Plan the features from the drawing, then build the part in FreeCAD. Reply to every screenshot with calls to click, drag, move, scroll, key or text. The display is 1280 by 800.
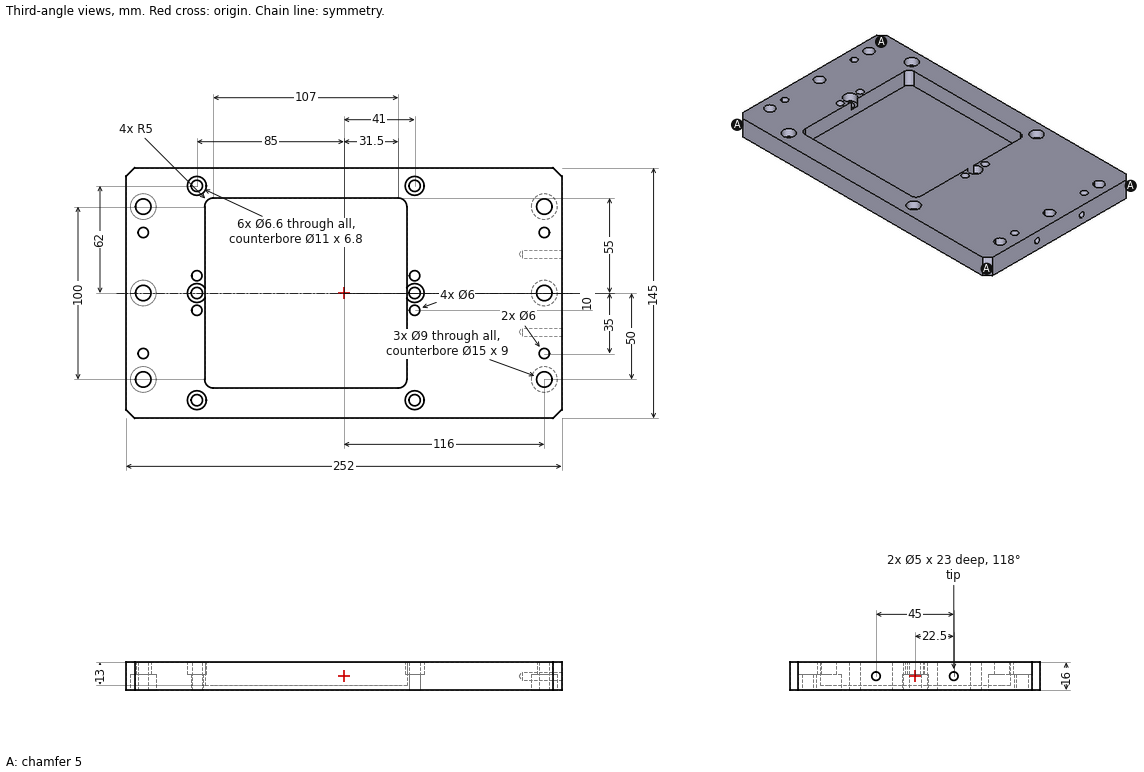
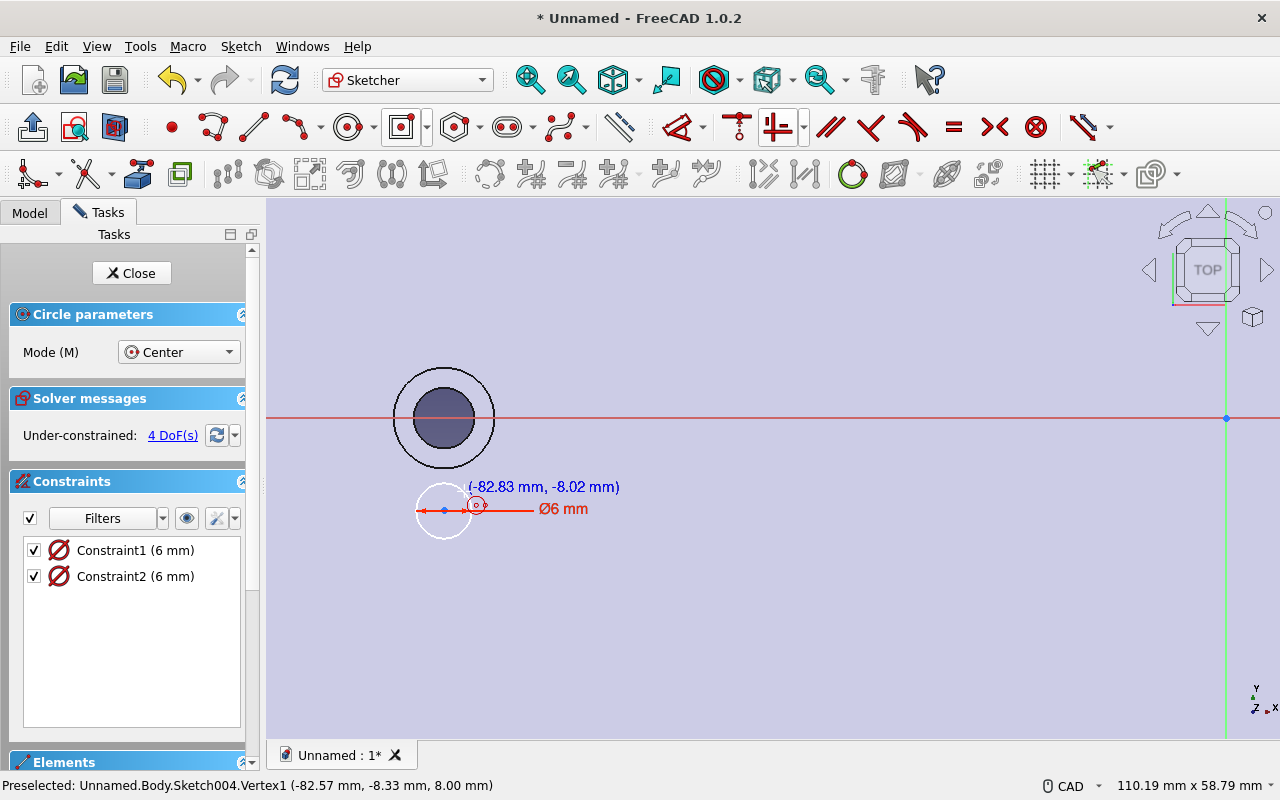
click(444, 326)
move(464, 307)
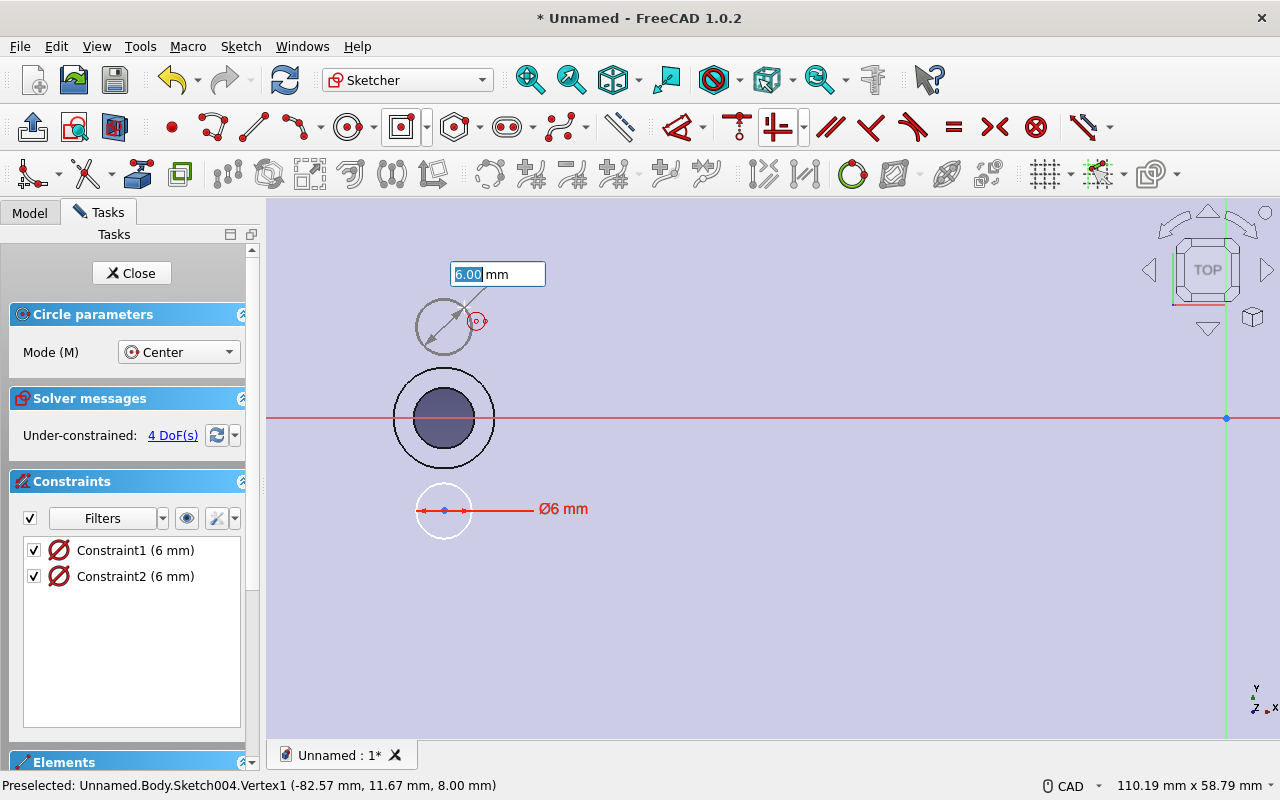
text(6)
key(Return)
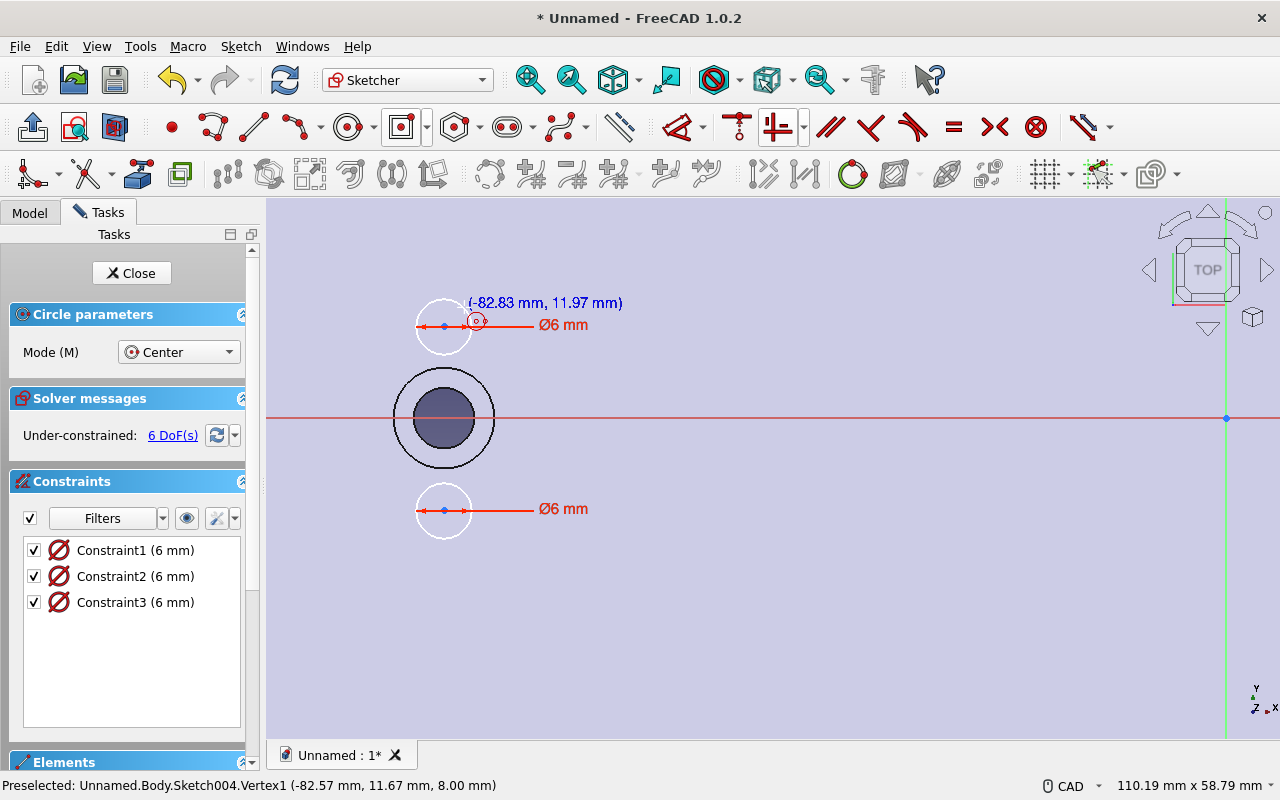
scroll(444, 510, down, 4)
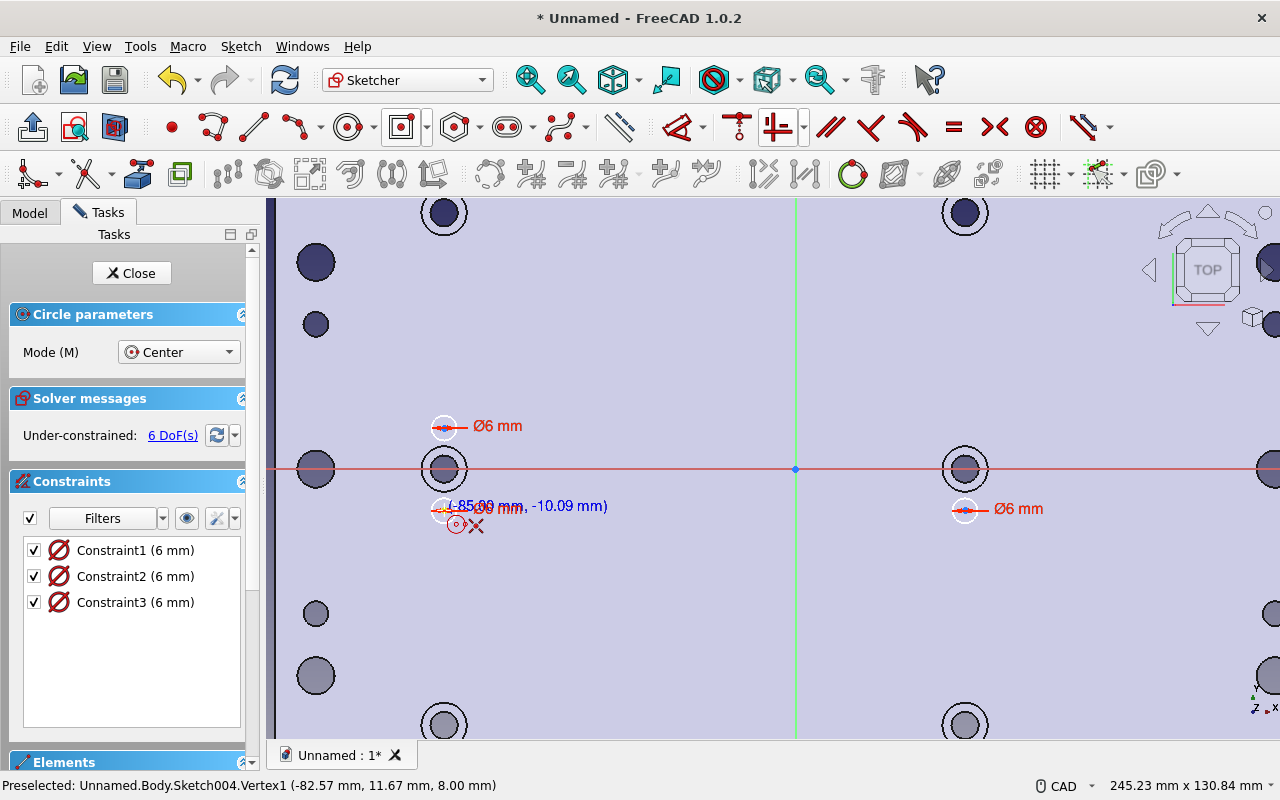
scroll(965, 428, up, 4)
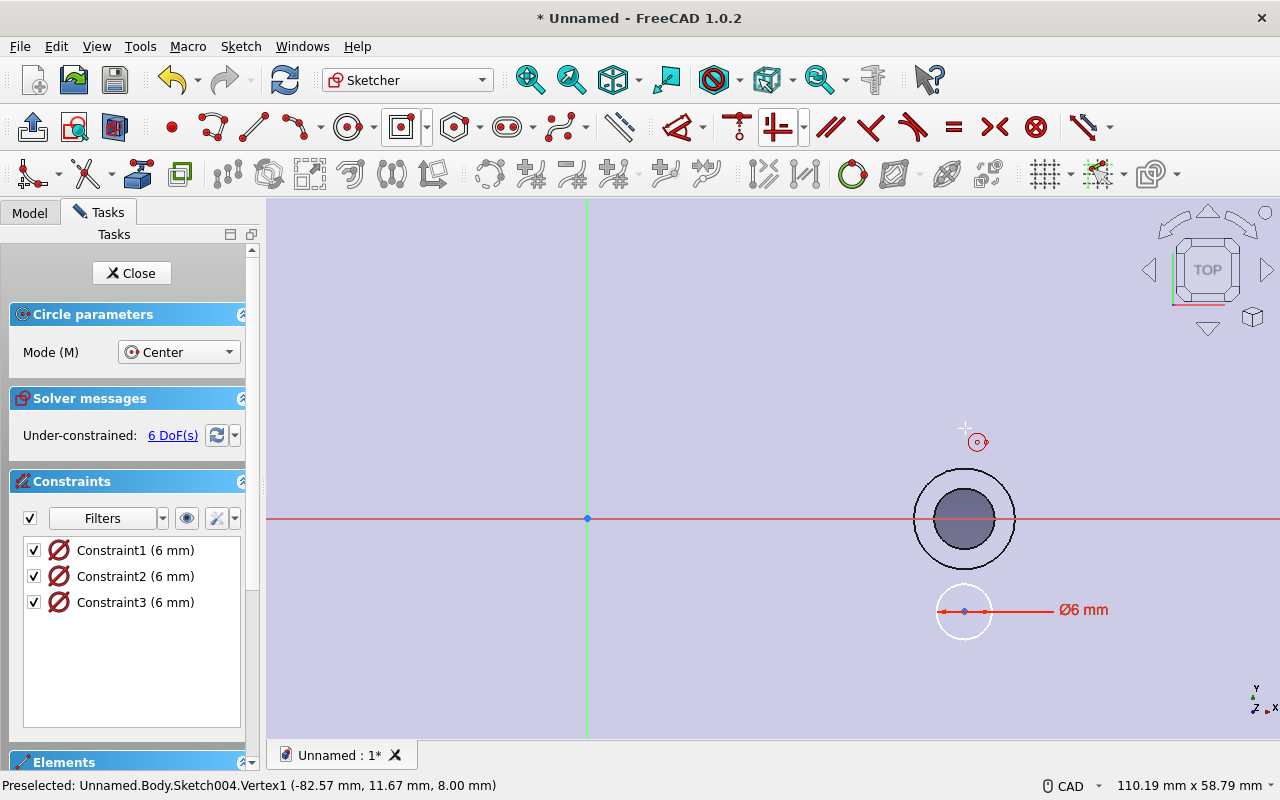
click(964, 427)
move(984, 407)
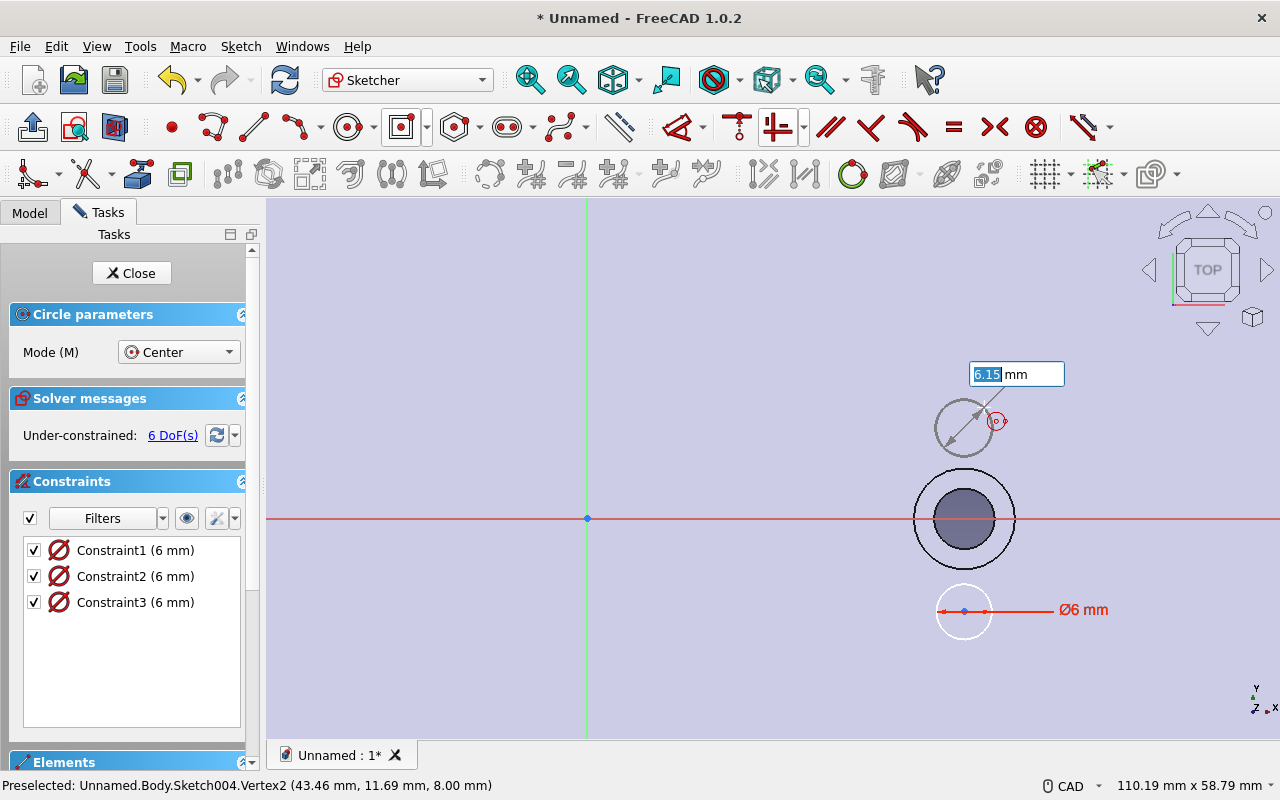
text(6)
key(Return)
key(Escape)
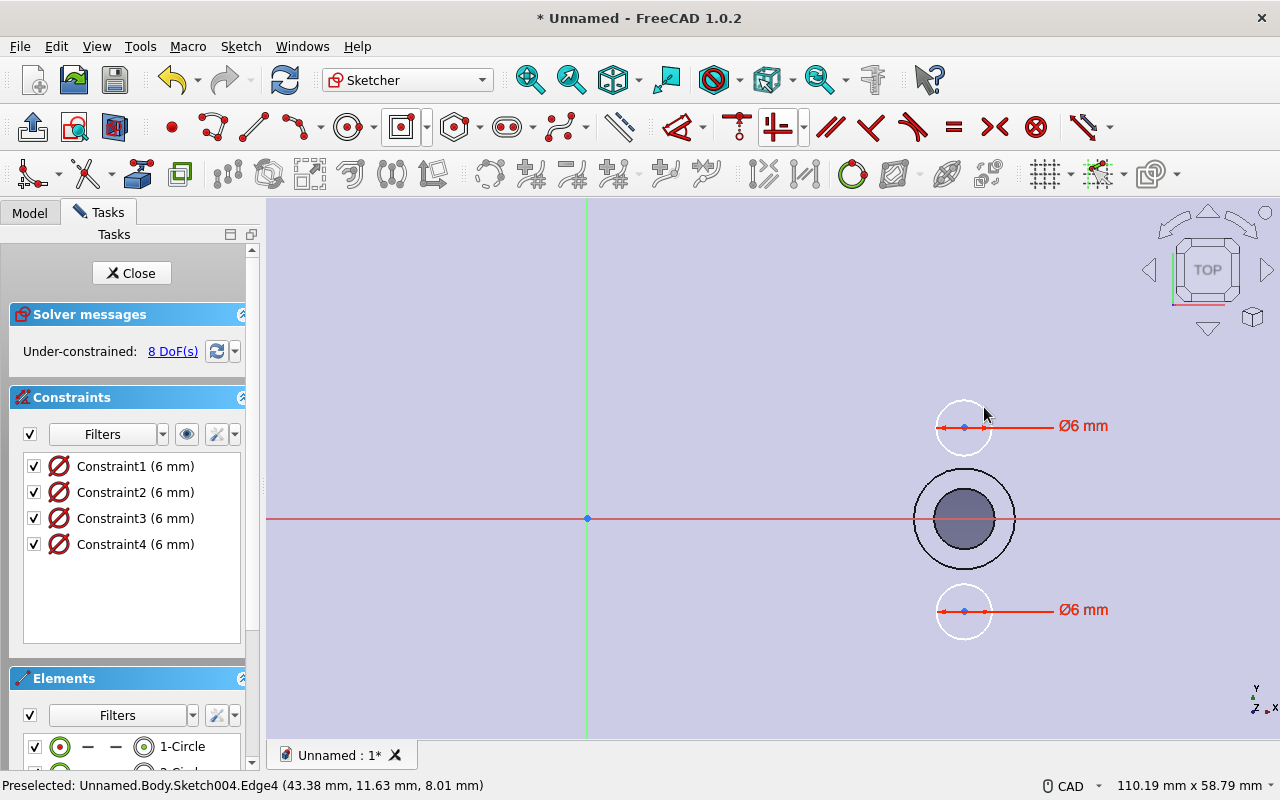
scroll(966, 427, down, 4)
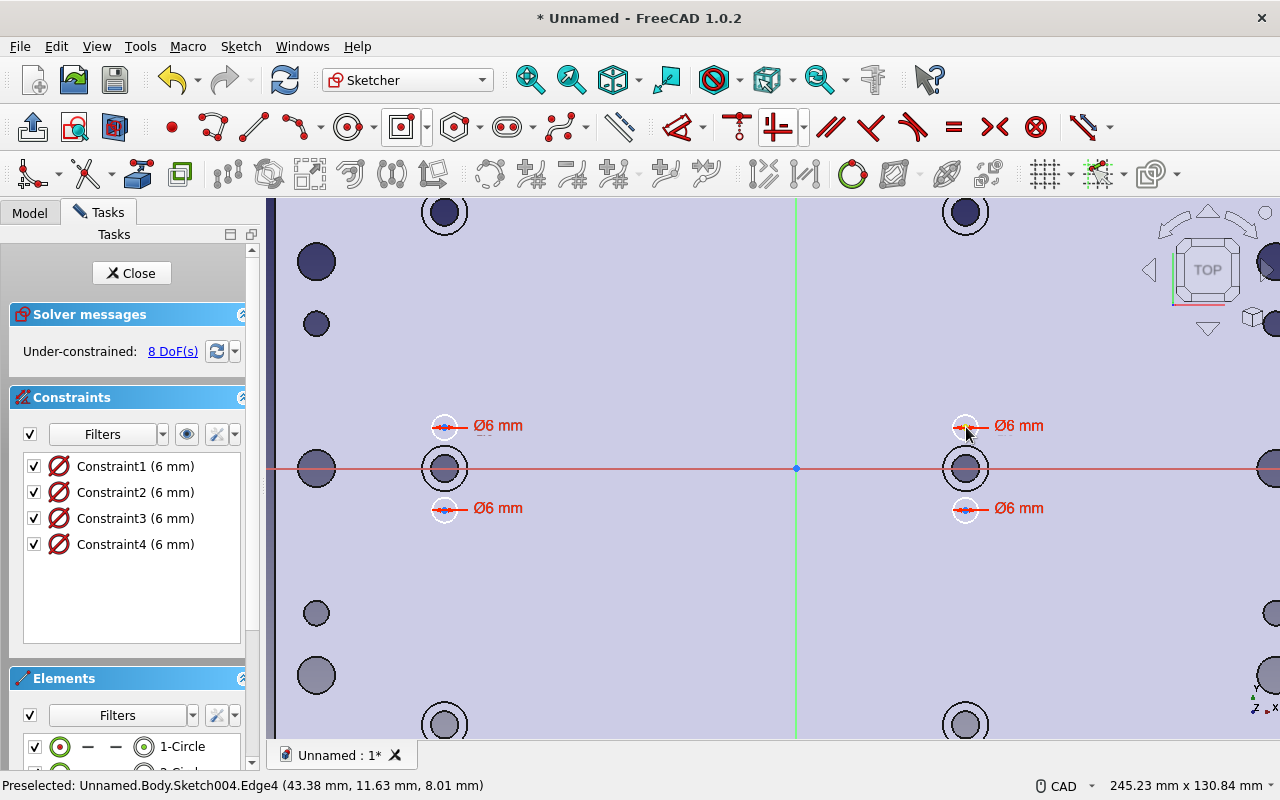
click(445, 510)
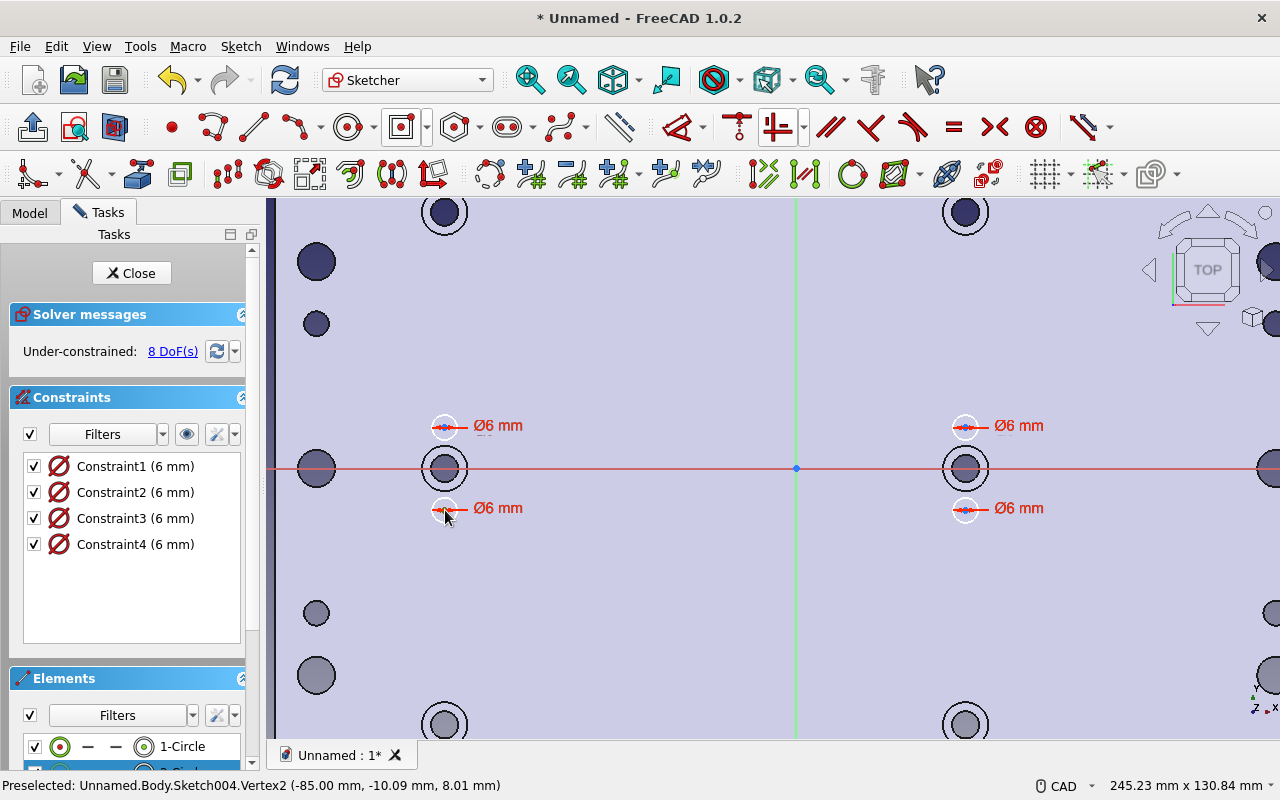
click(445, 428)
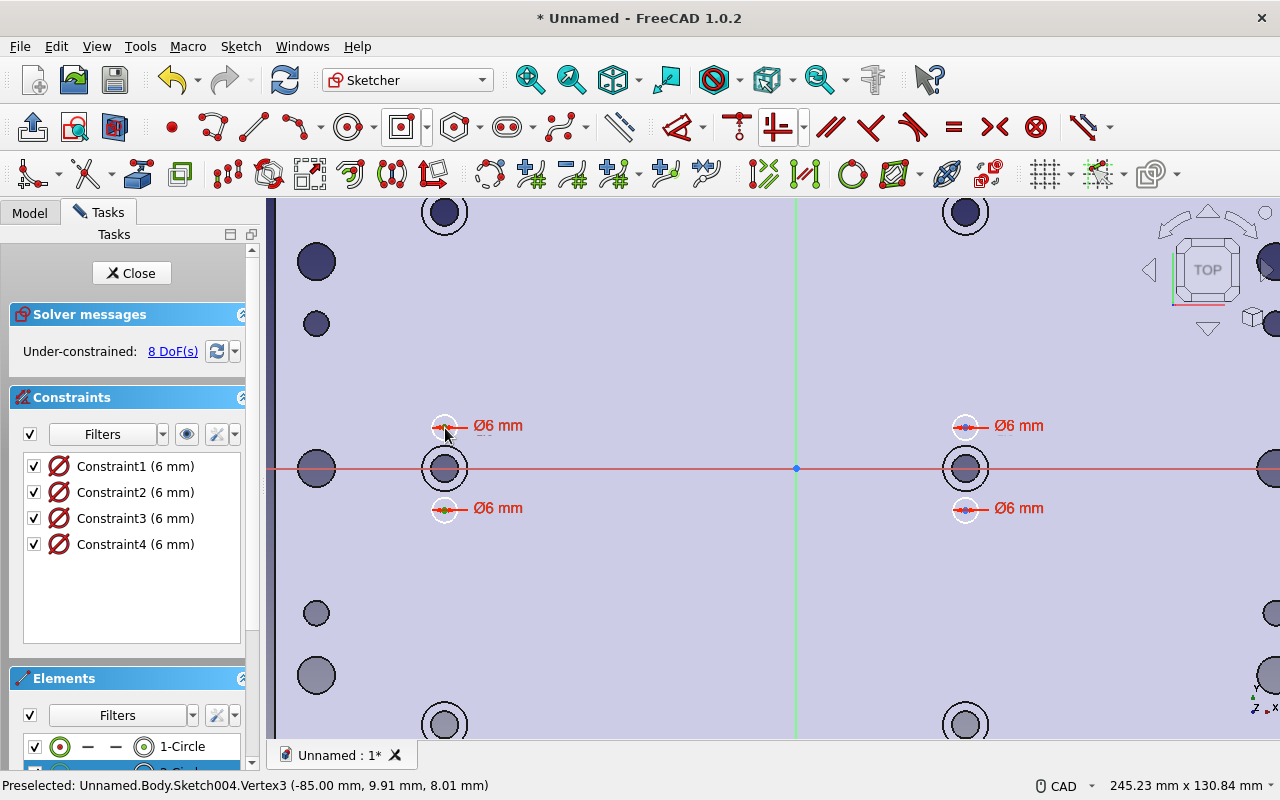
click(353, 468)